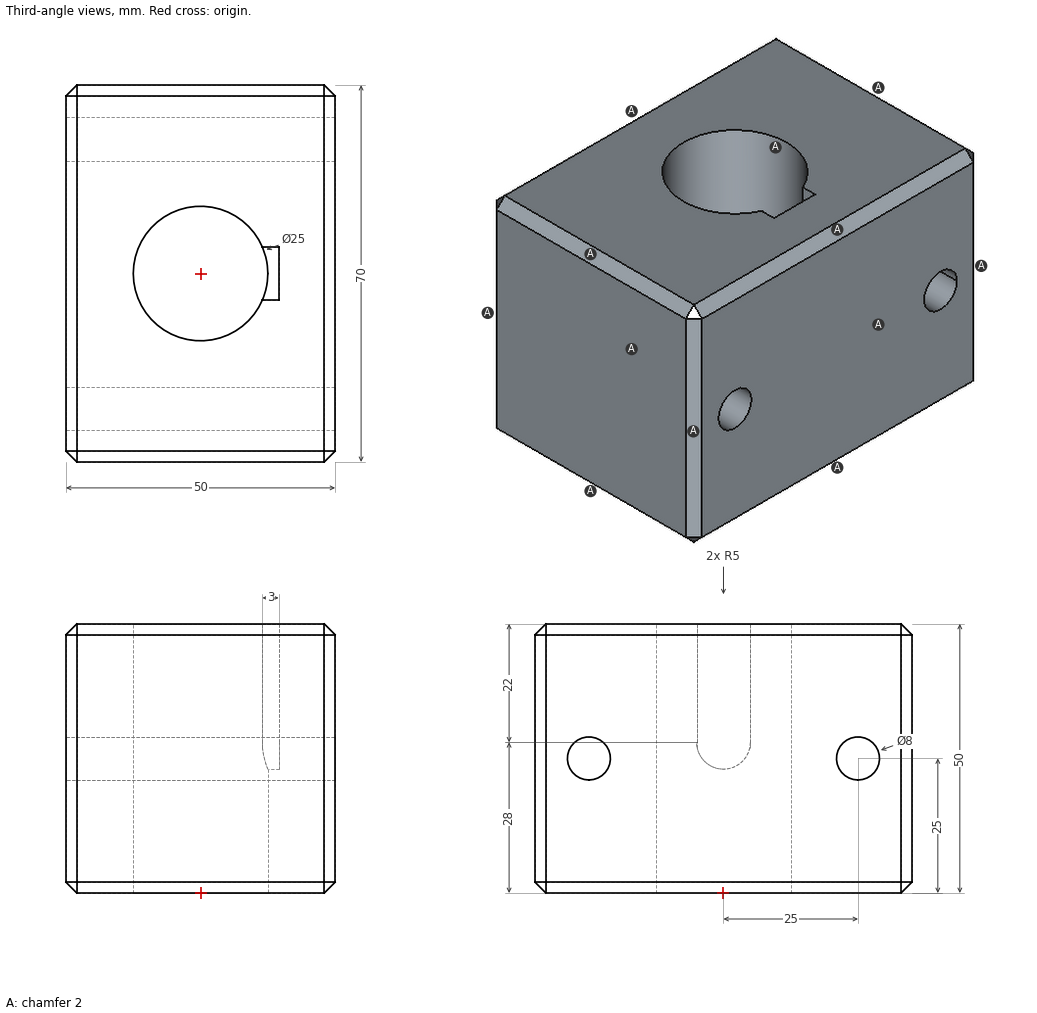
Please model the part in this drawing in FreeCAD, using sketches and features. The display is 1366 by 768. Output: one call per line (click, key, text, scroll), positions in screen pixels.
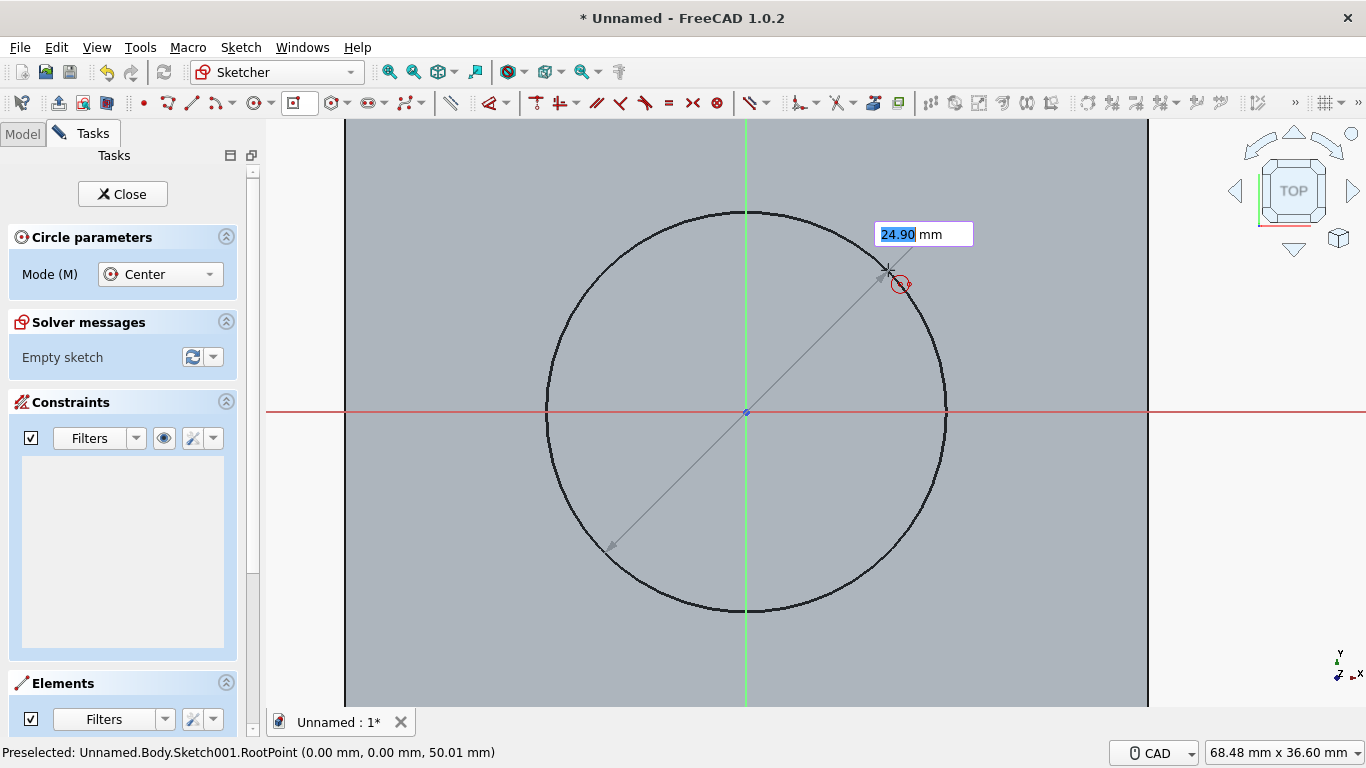
text(25)
key(Return)
key(Escape)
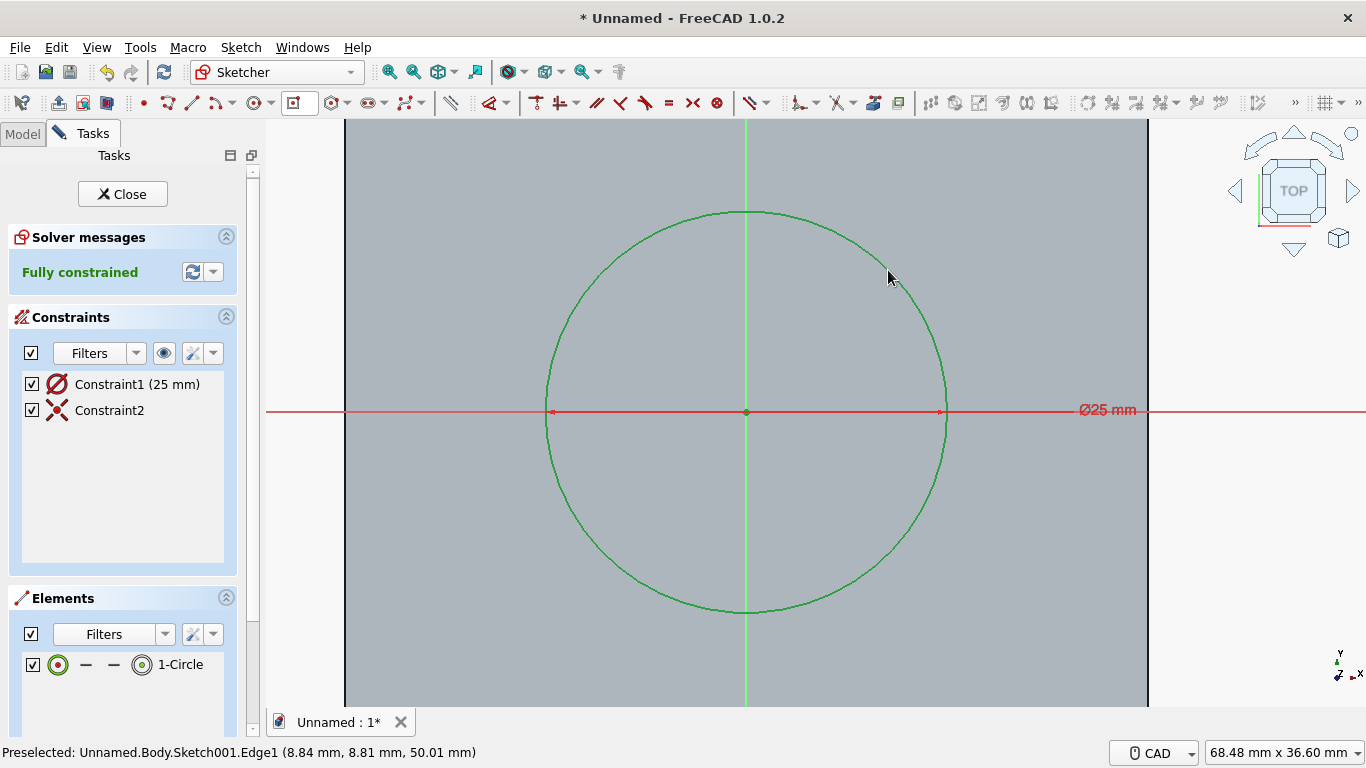
click(123, 194)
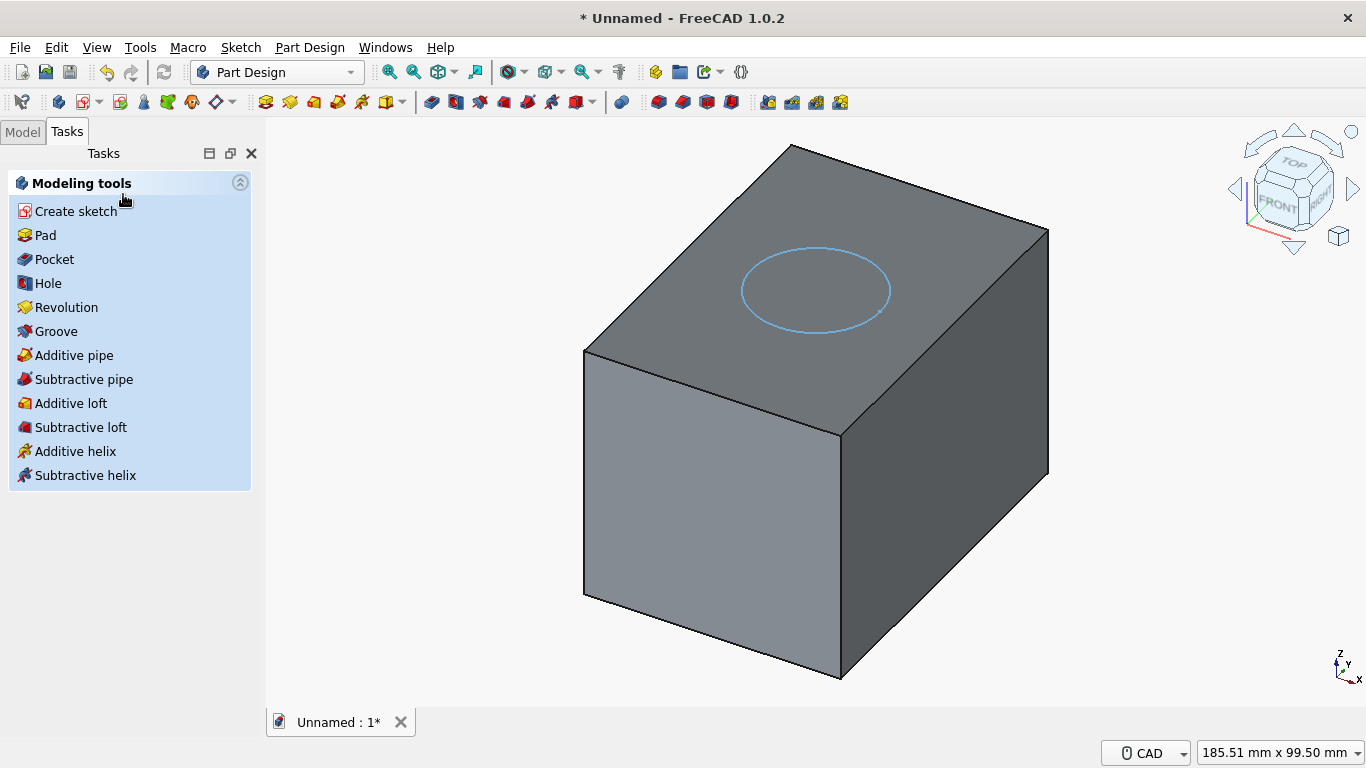
click(432, 102)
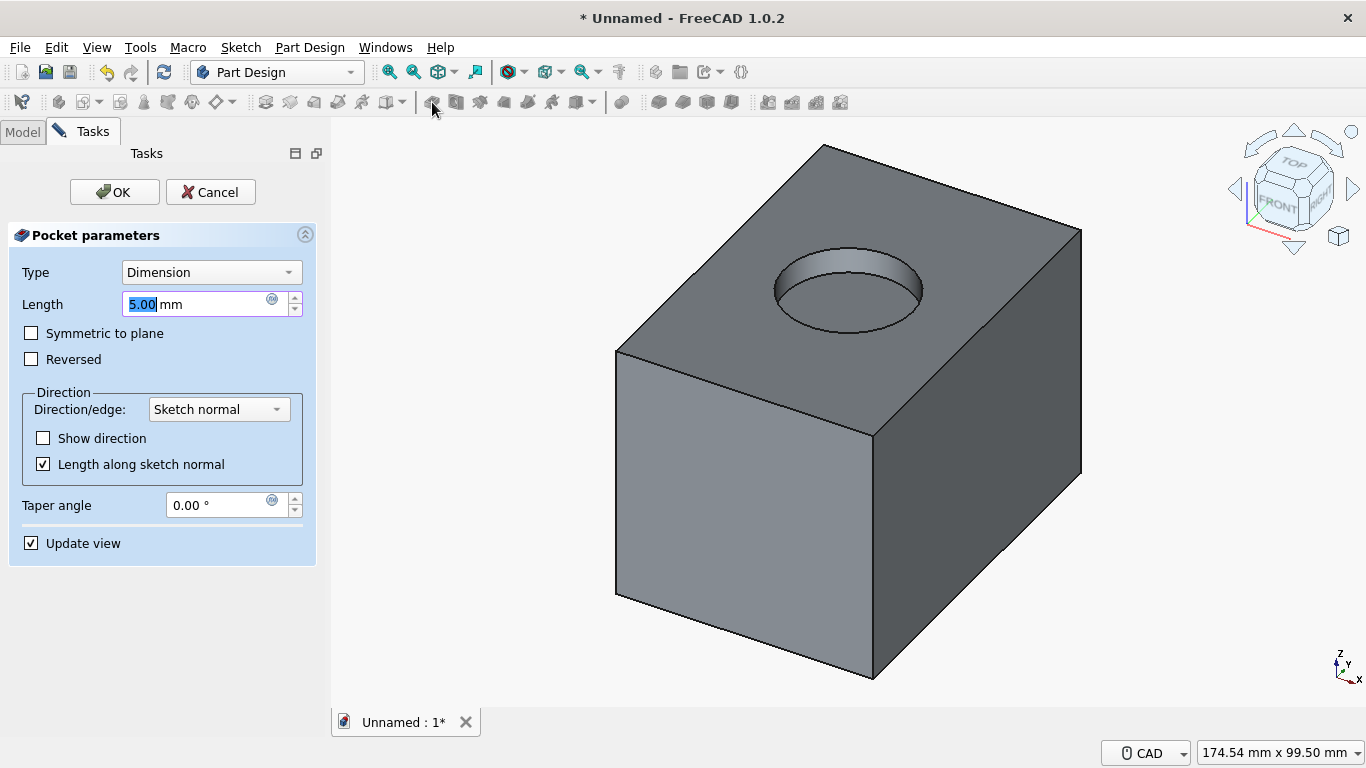
click(212, 272)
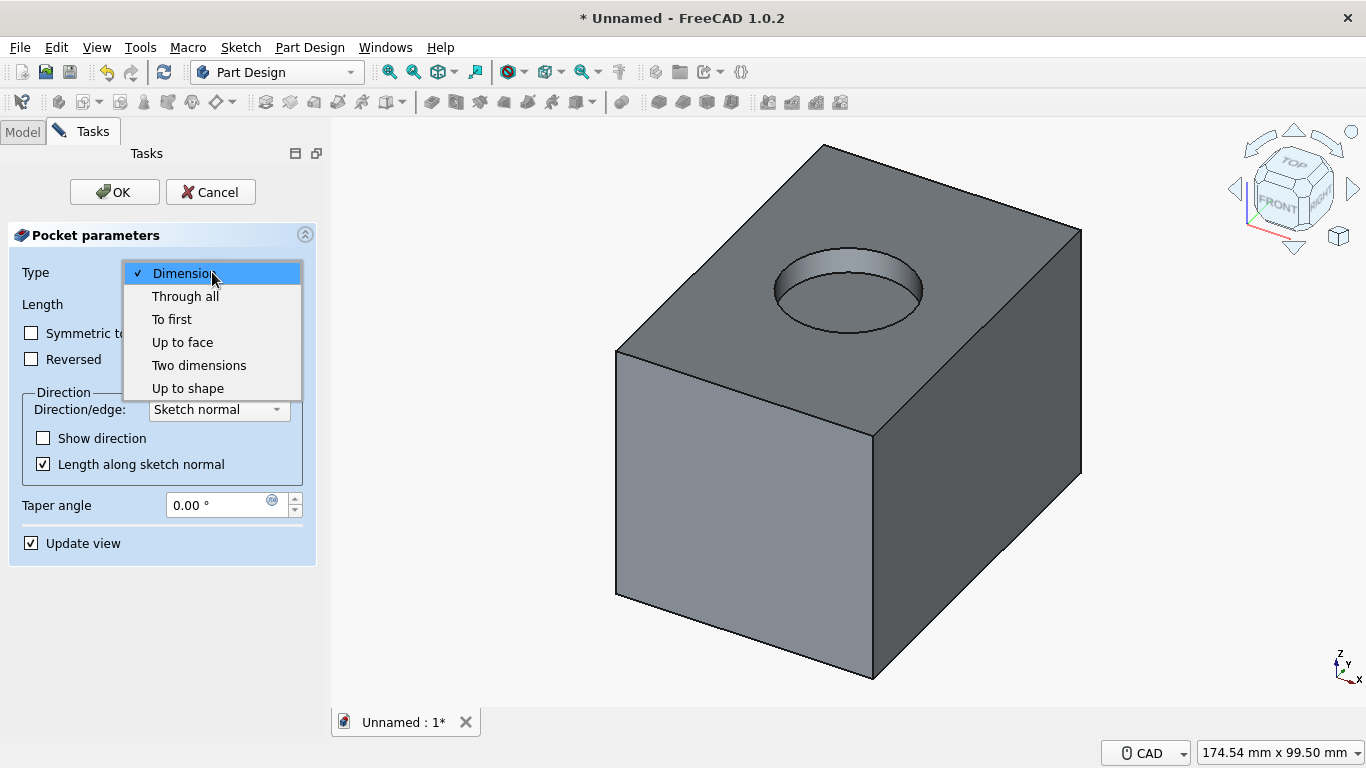
click(212, 296)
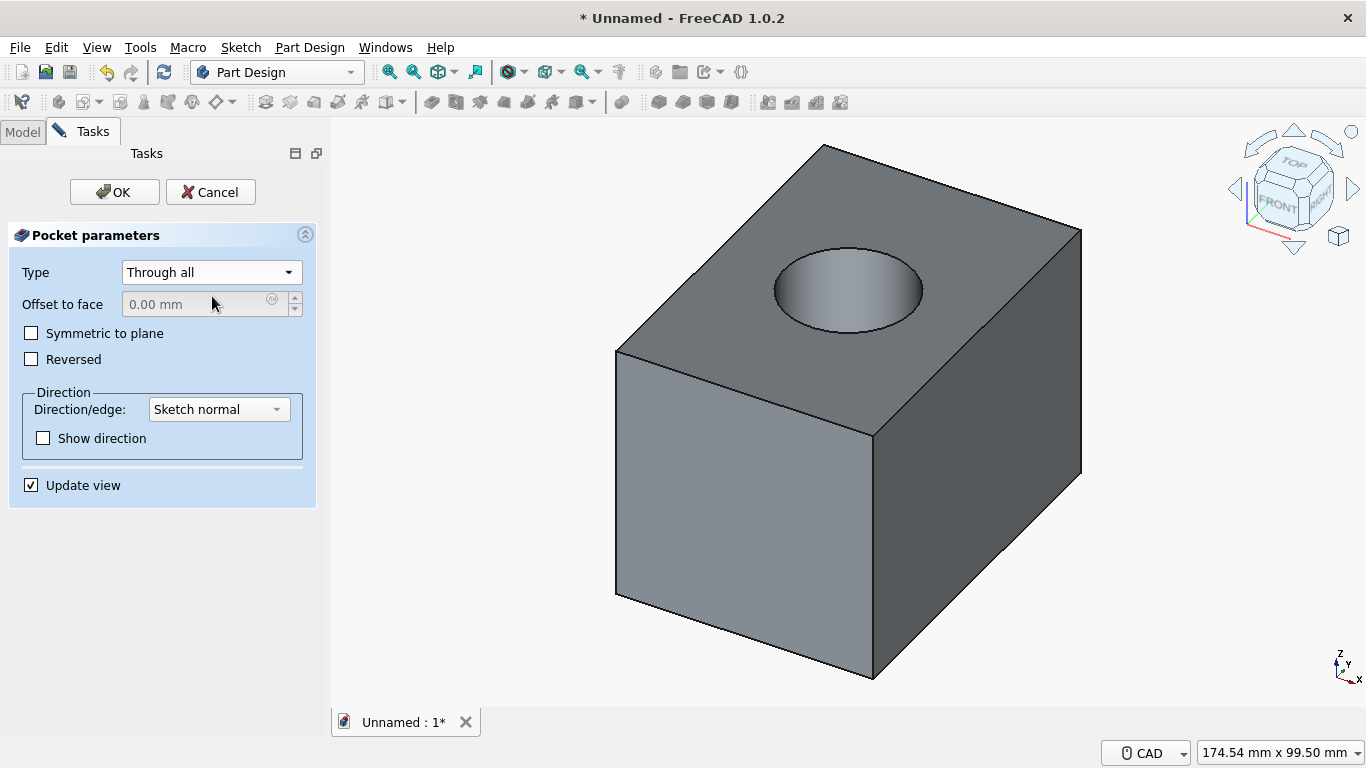
click(115, 192)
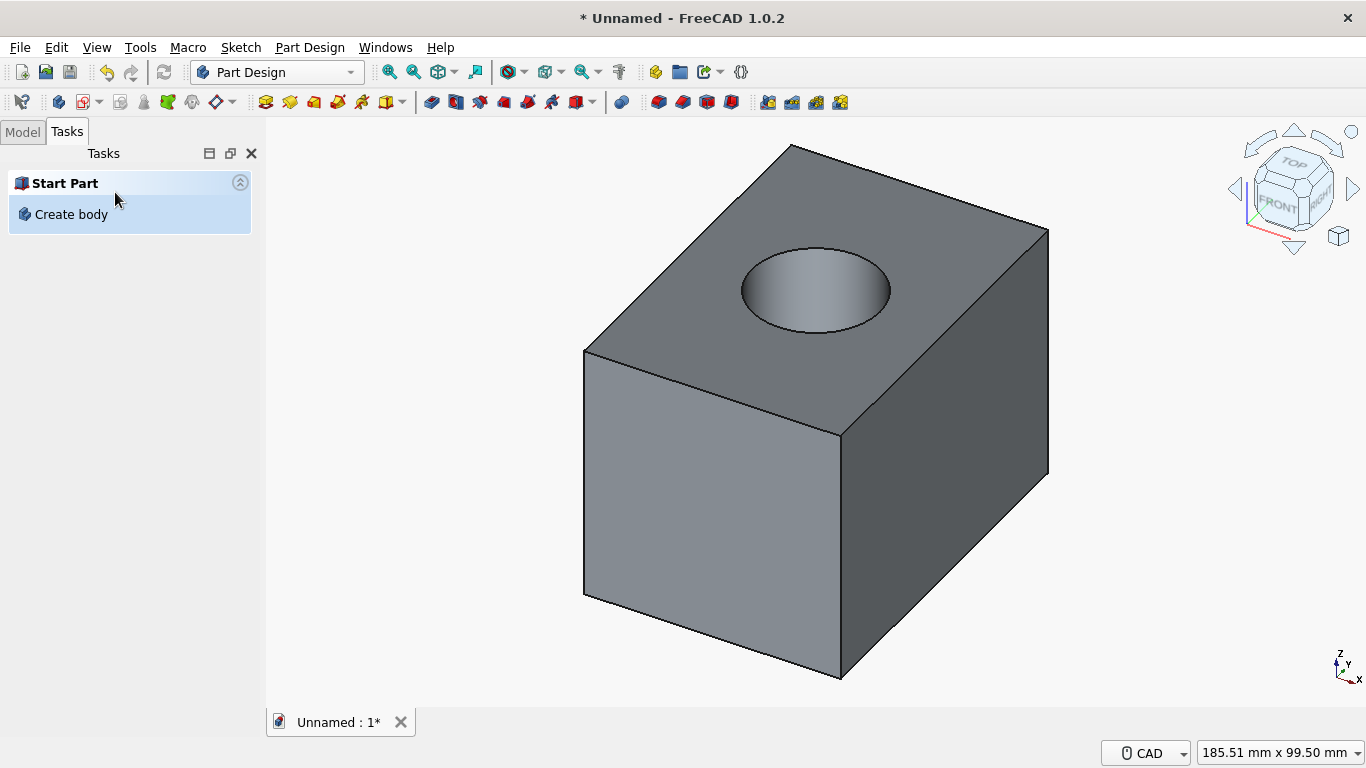
click(974, 424)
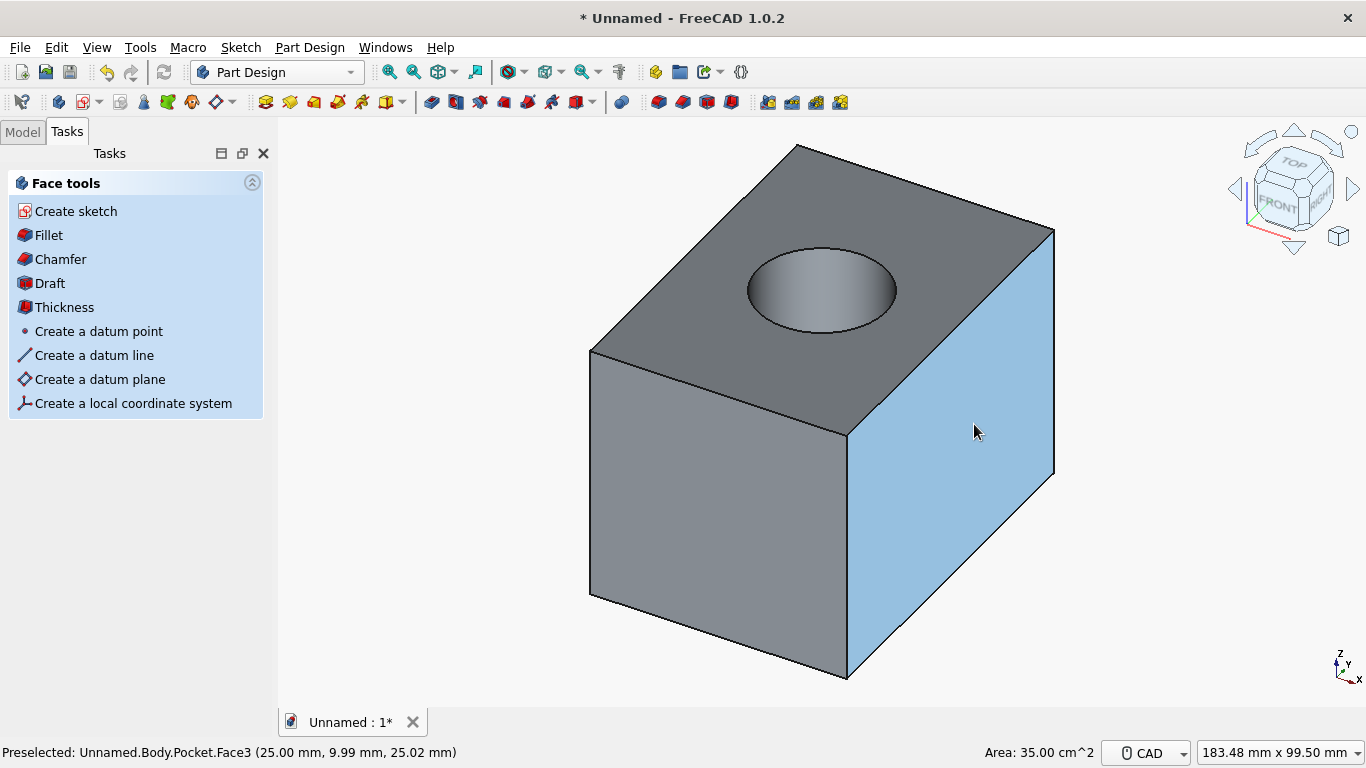
click(84, 102)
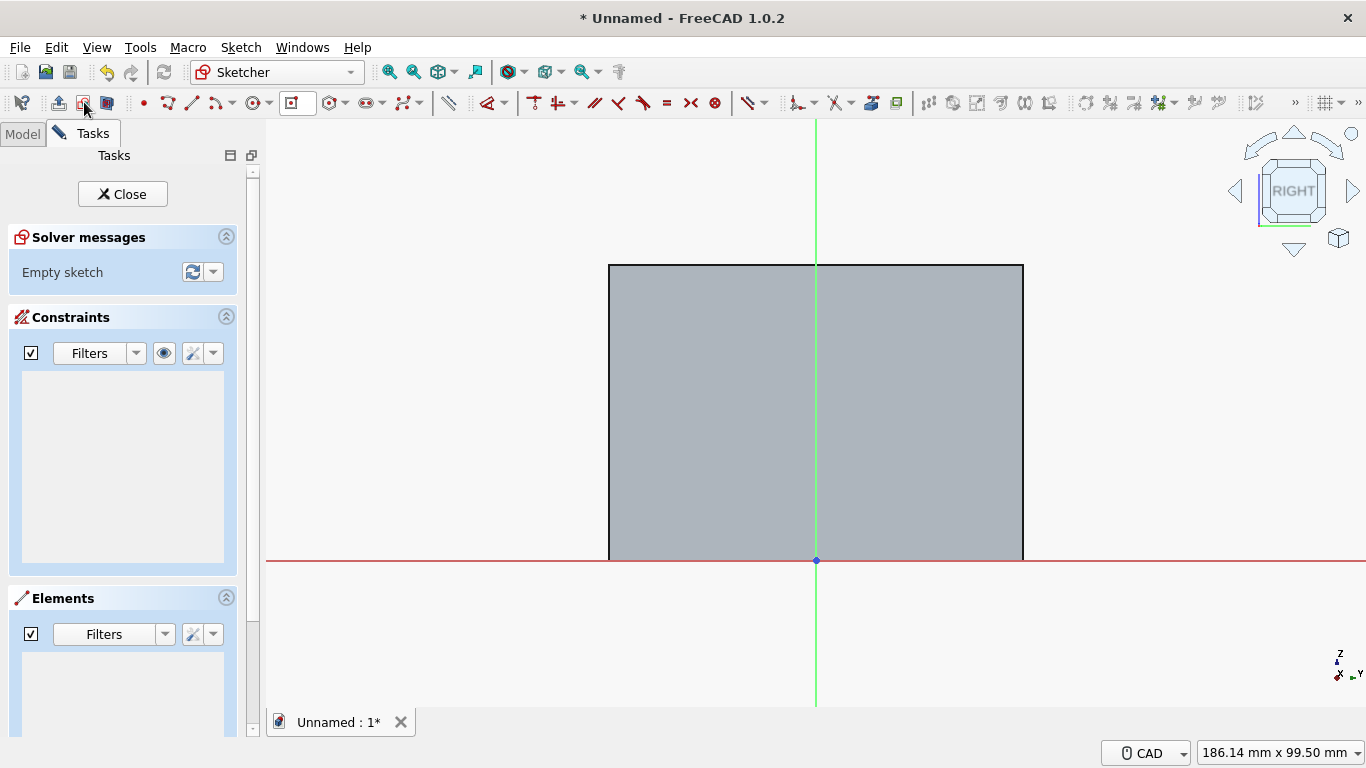
scroll(998, 413, up, 10)